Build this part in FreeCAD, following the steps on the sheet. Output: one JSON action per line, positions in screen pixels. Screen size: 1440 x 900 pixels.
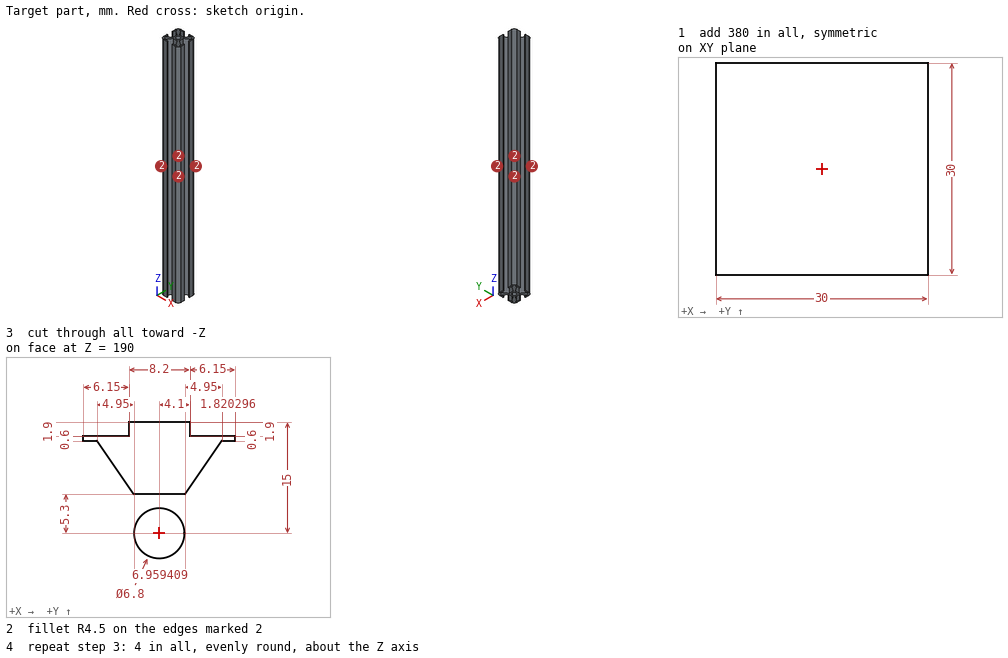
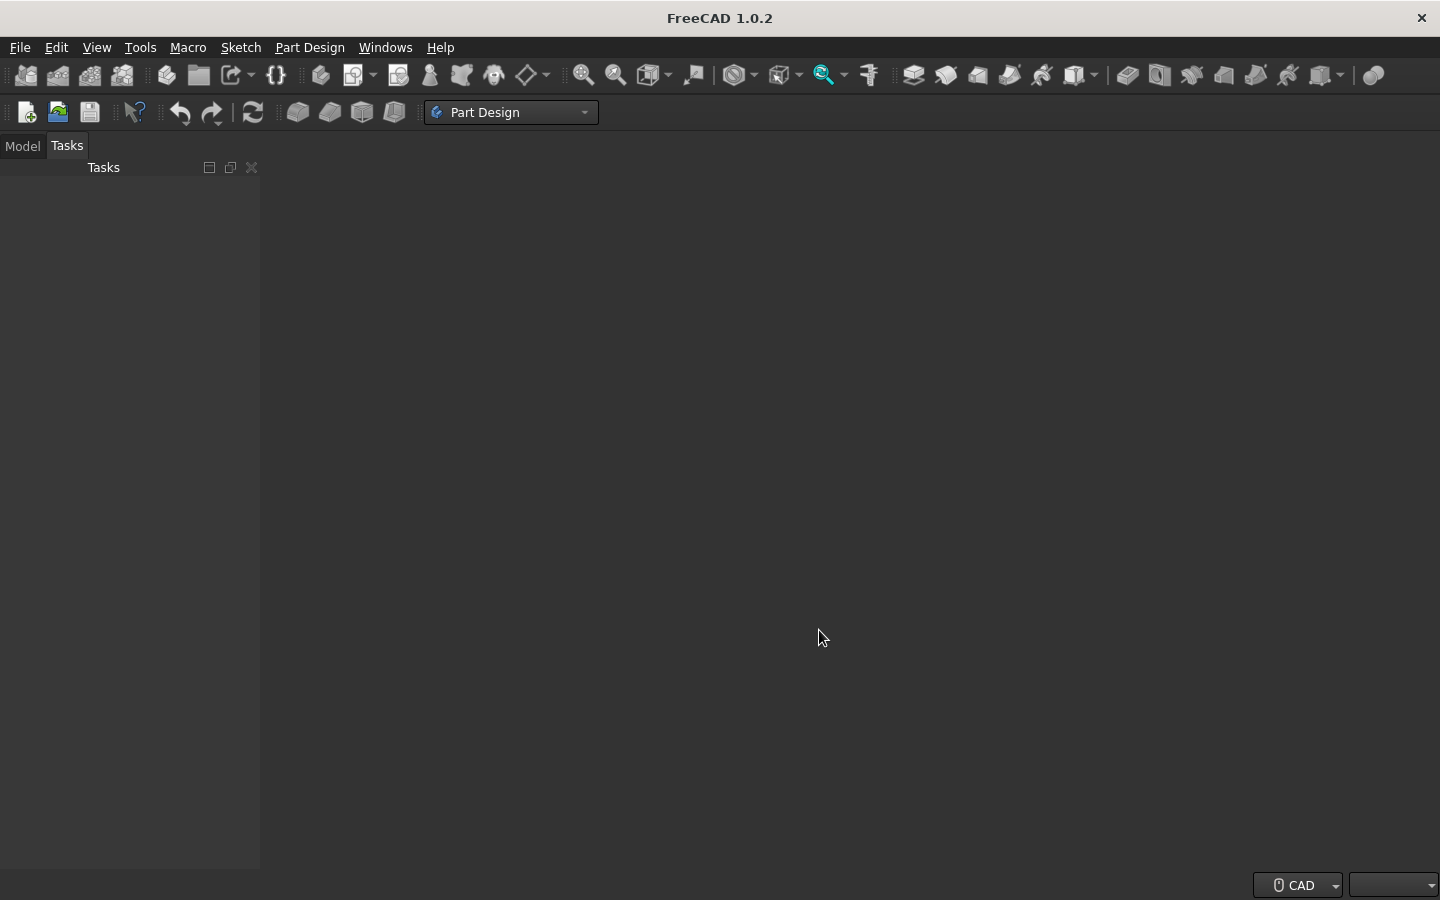
{"action": "left_click", "coordinate": [26, 112]}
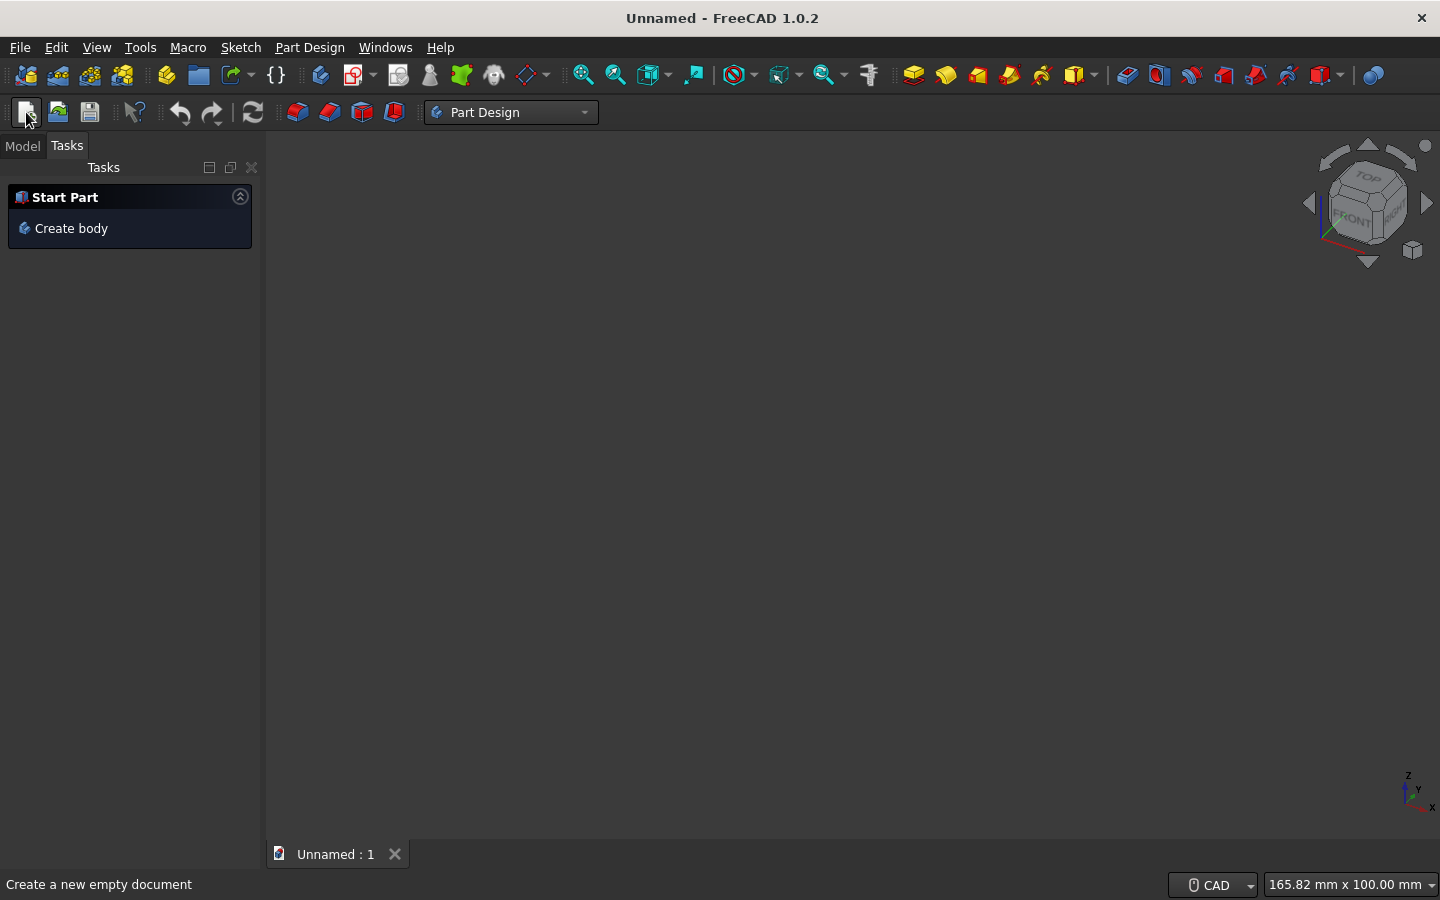
{"action": "left_click", "coordinate": [354, 76]}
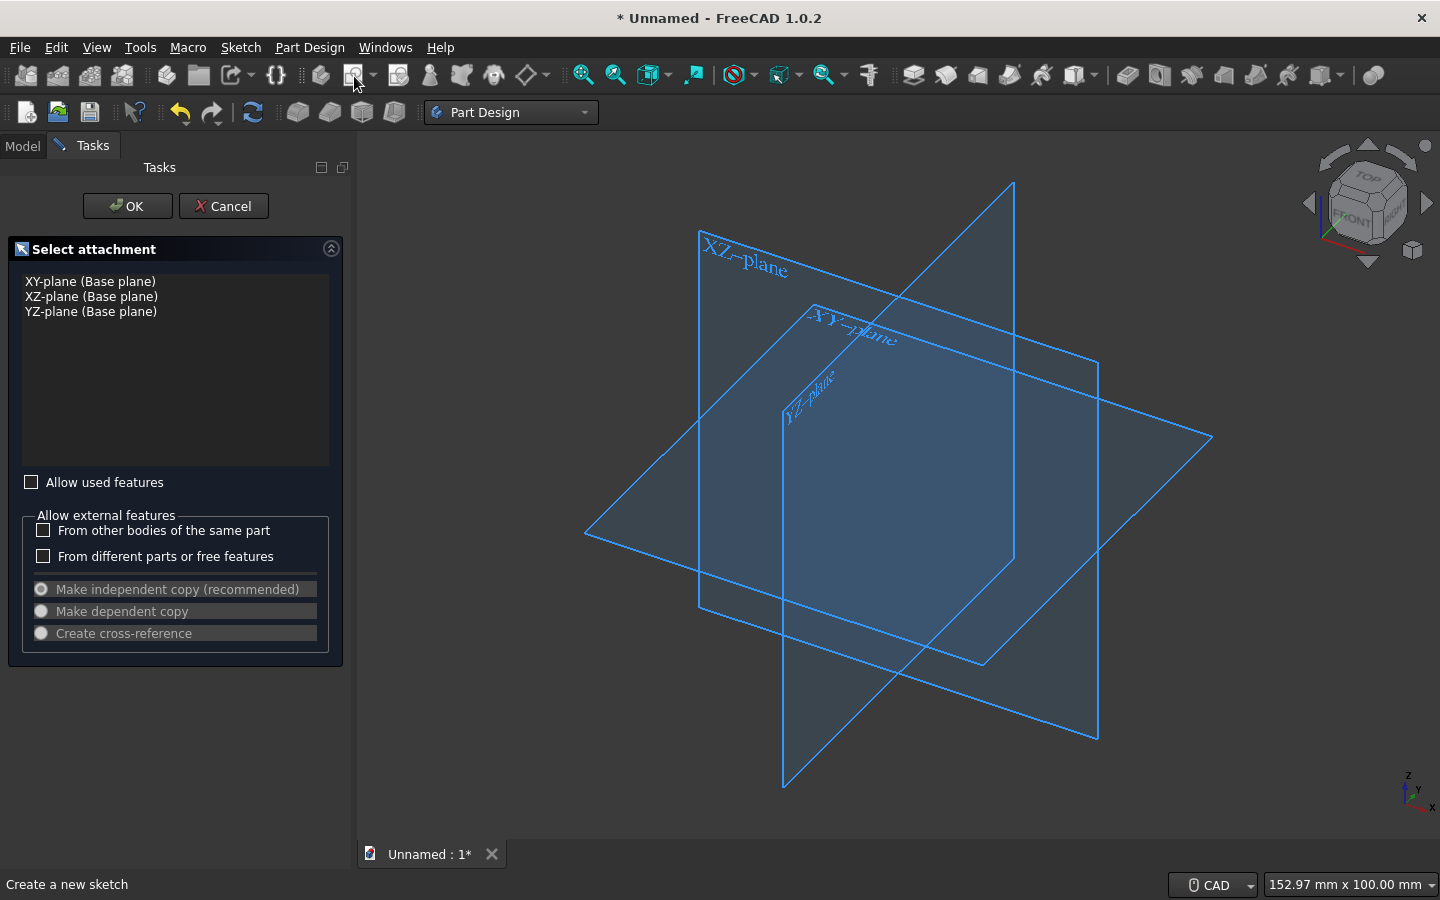
{"action": "left_click", "coordinate": [82, 282]}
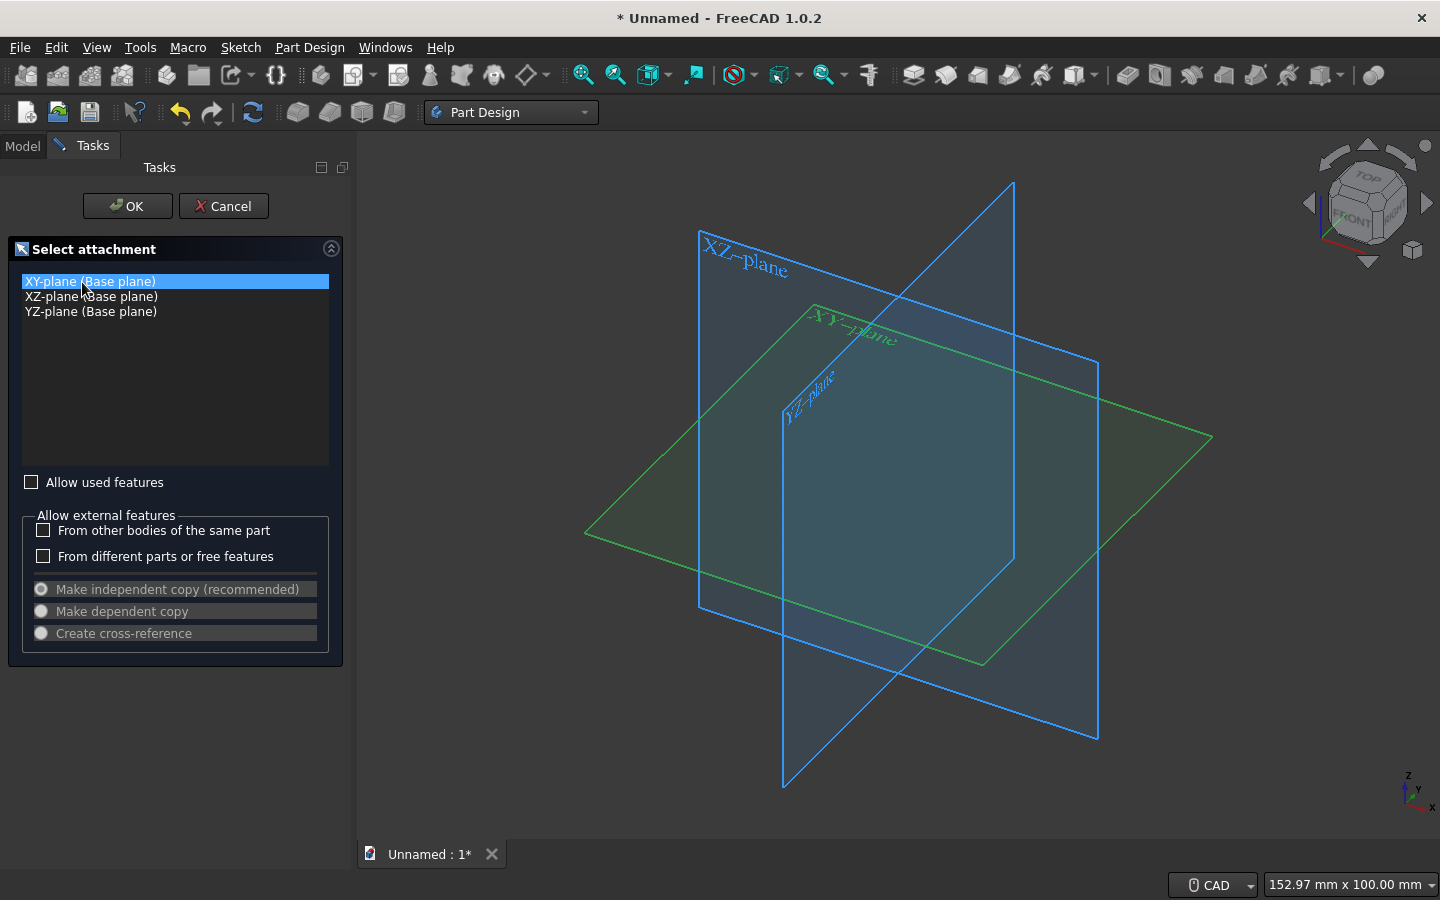
{"action": "left_click", "coordinate": [128, 206]}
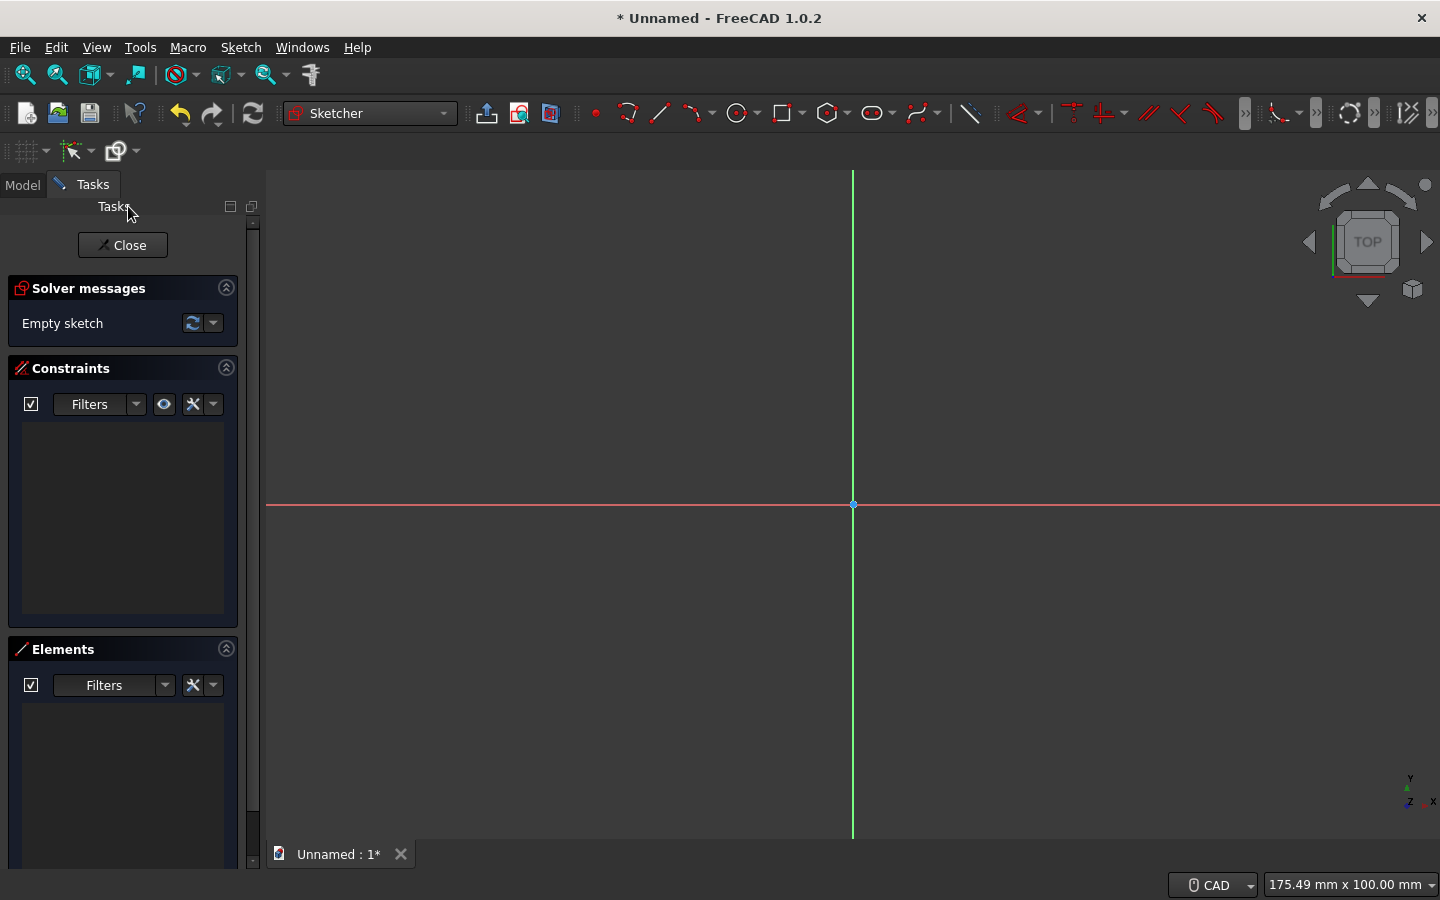
{"action": "scroll", "coordinate": [909, 504], "scroll_direction": "up", "scroll_amount": 4}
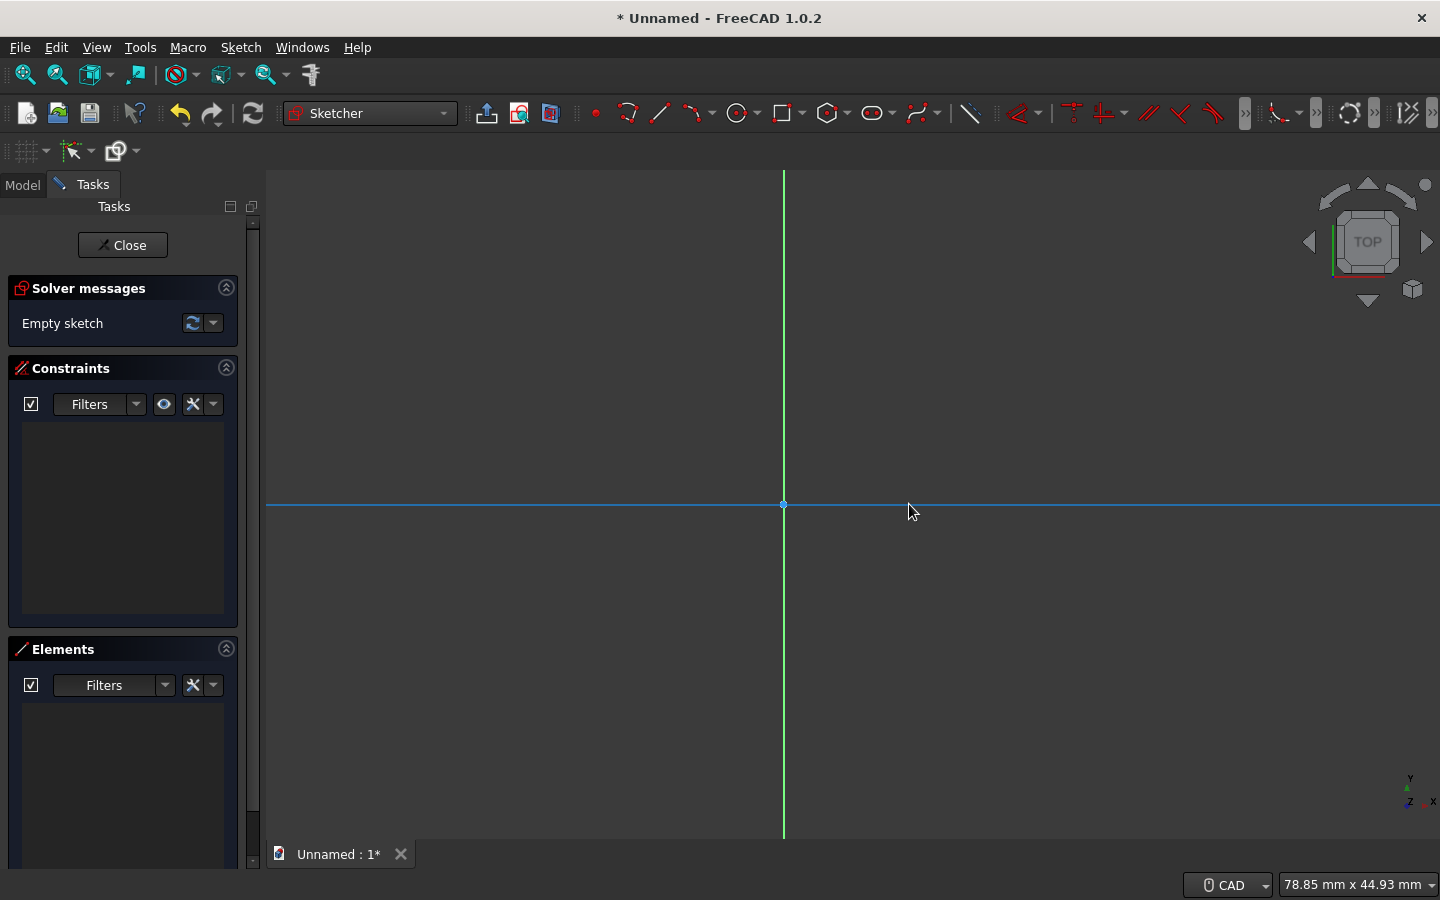
{"action": "left_click", "coordinate": [804, 114]}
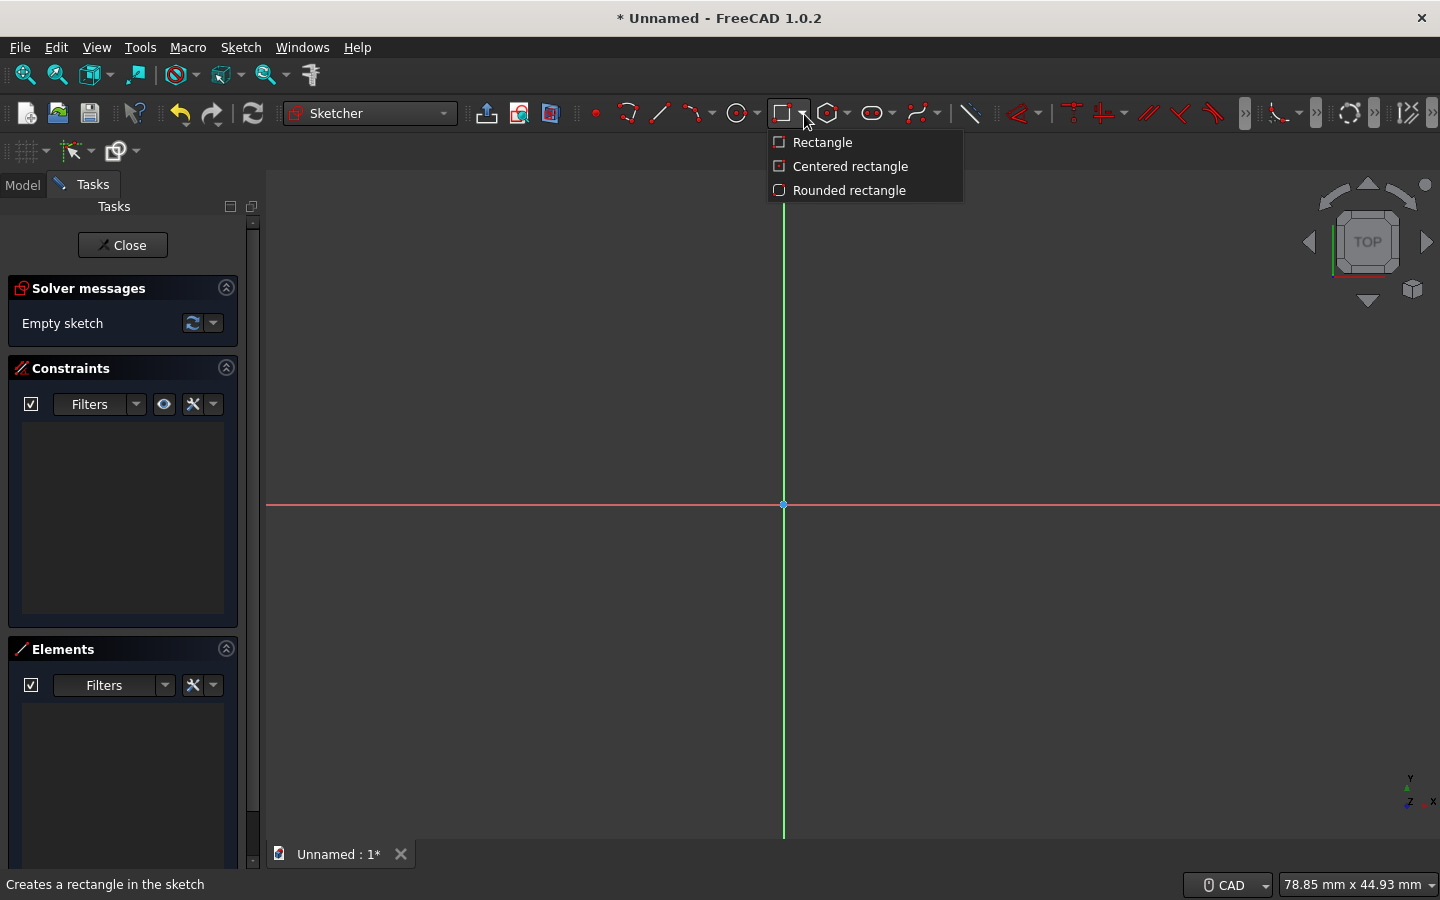
{"action": "left_click", "coordinate": [866, 166]}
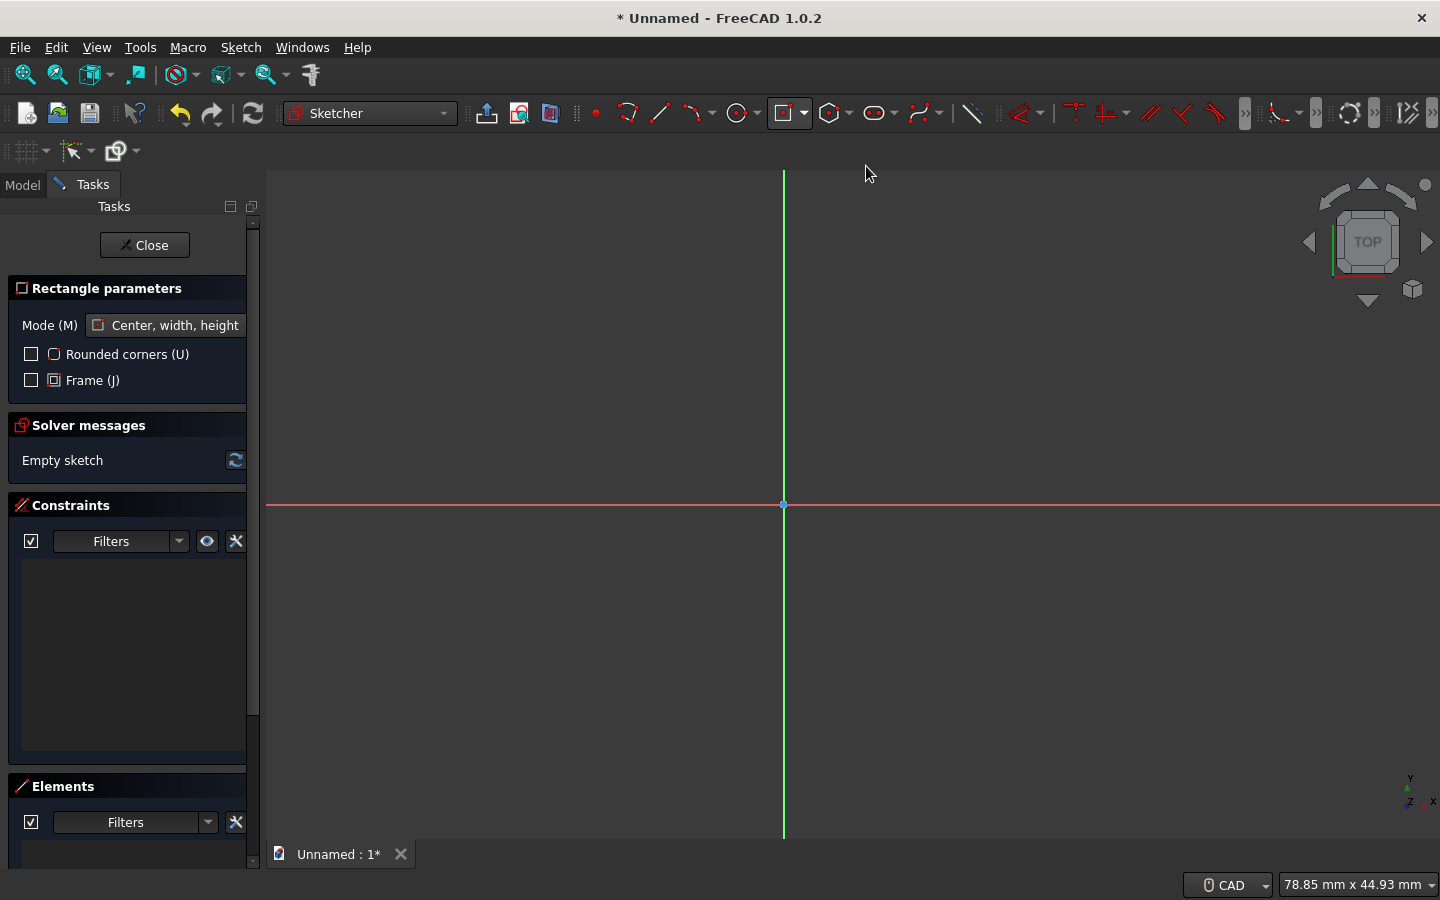
{"action": "left_click", "coordinate": [784, 504]}
{"action": "left_click", "coordinate": [1007, 281]}
{"action": "key", "text": "Escape"}